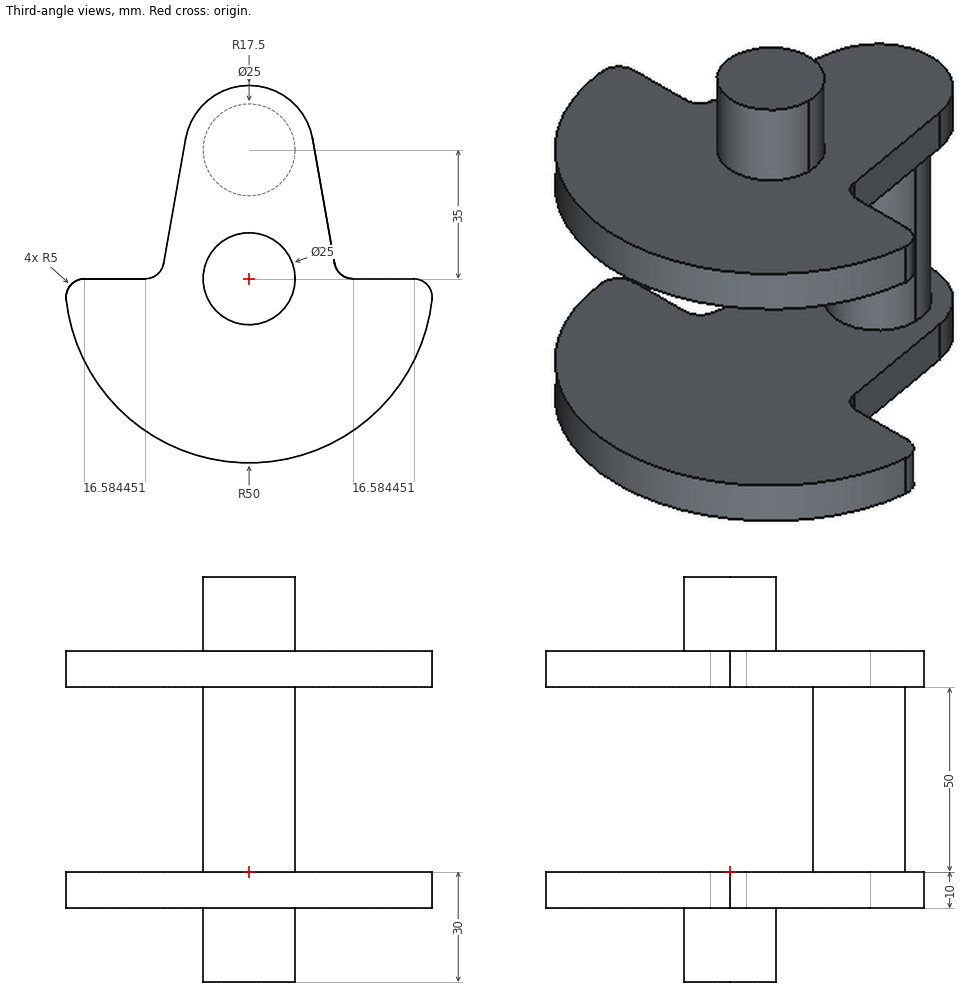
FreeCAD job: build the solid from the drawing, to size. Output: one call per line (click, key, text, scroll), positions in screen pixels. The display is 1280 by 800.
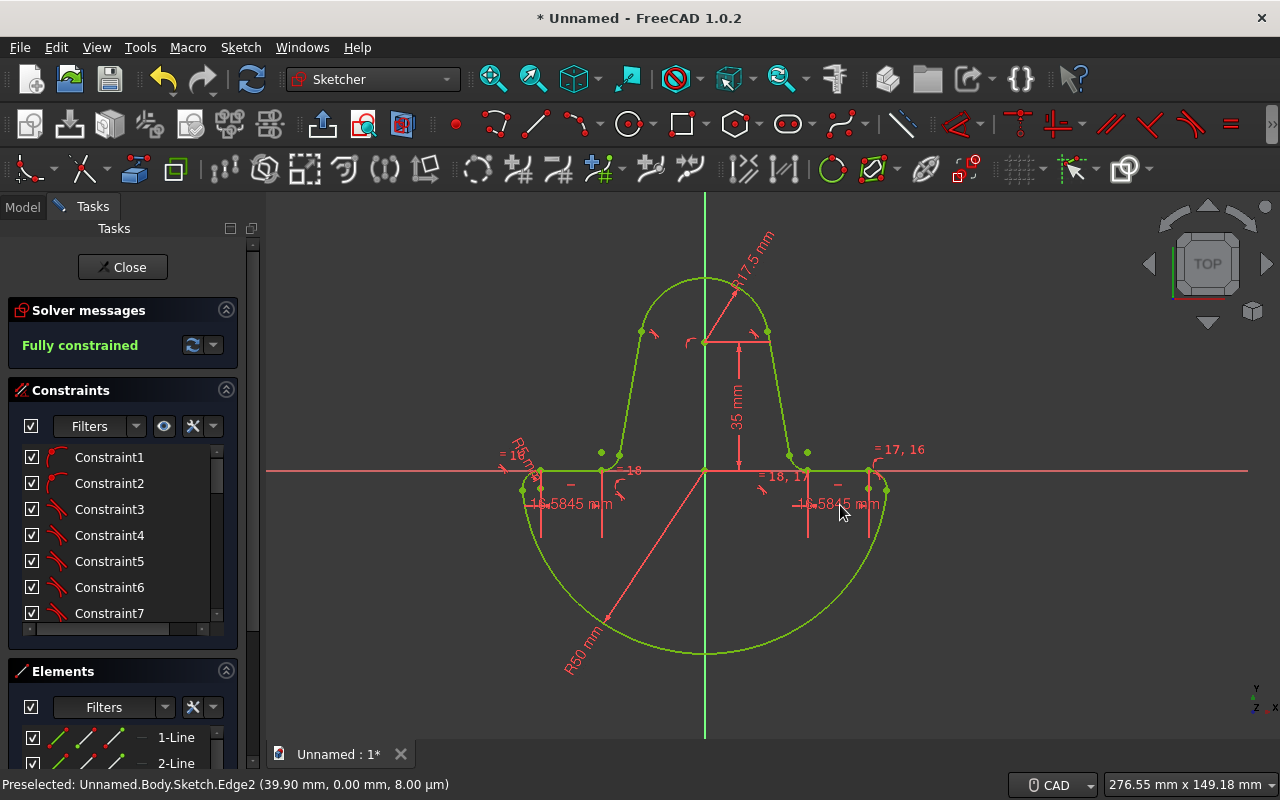
click(123, 267)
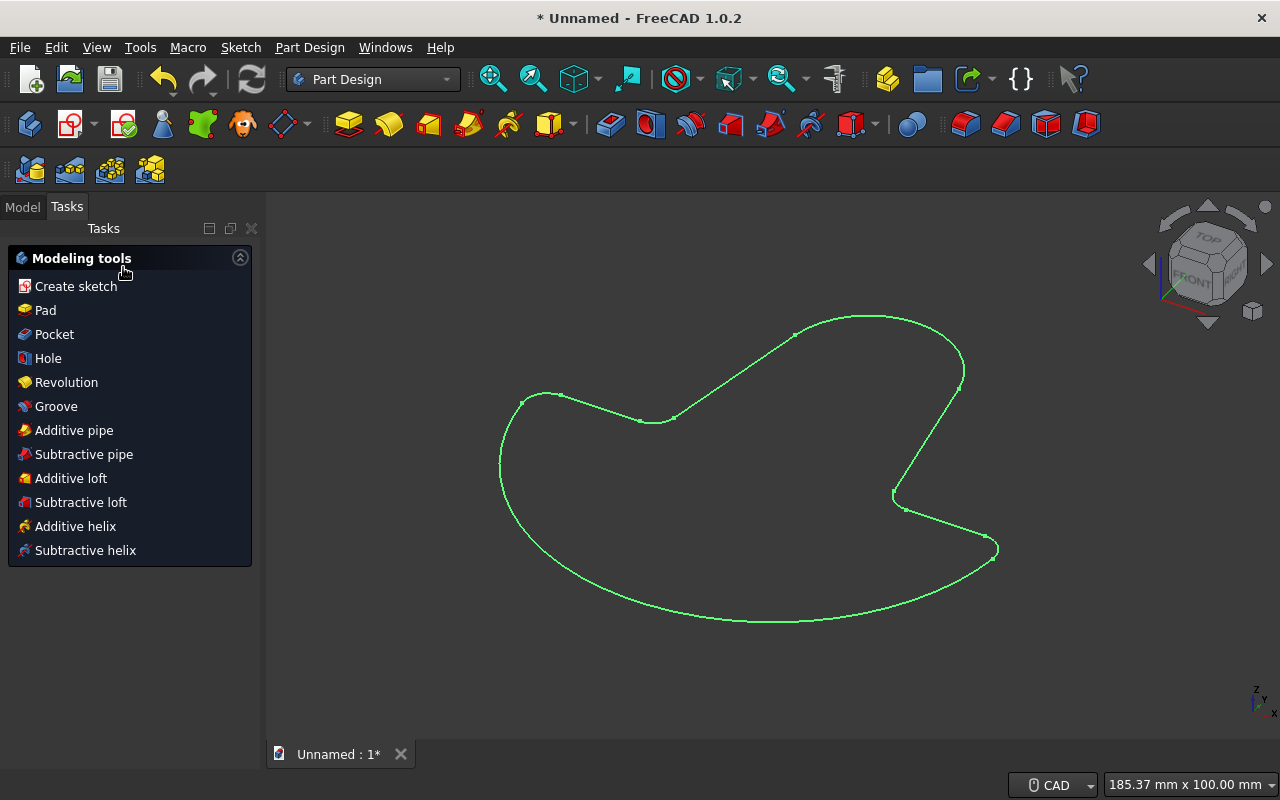
click(350, 124)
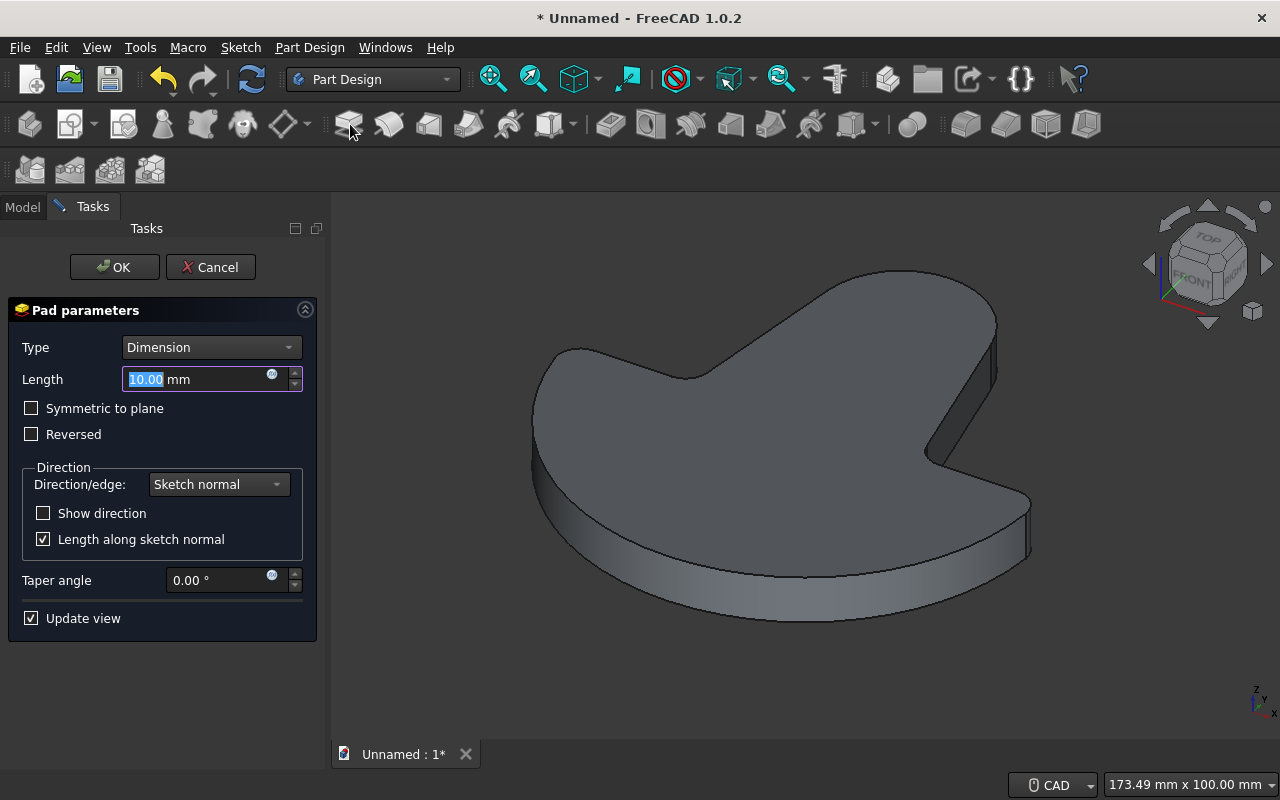
text(10)
key(Tab)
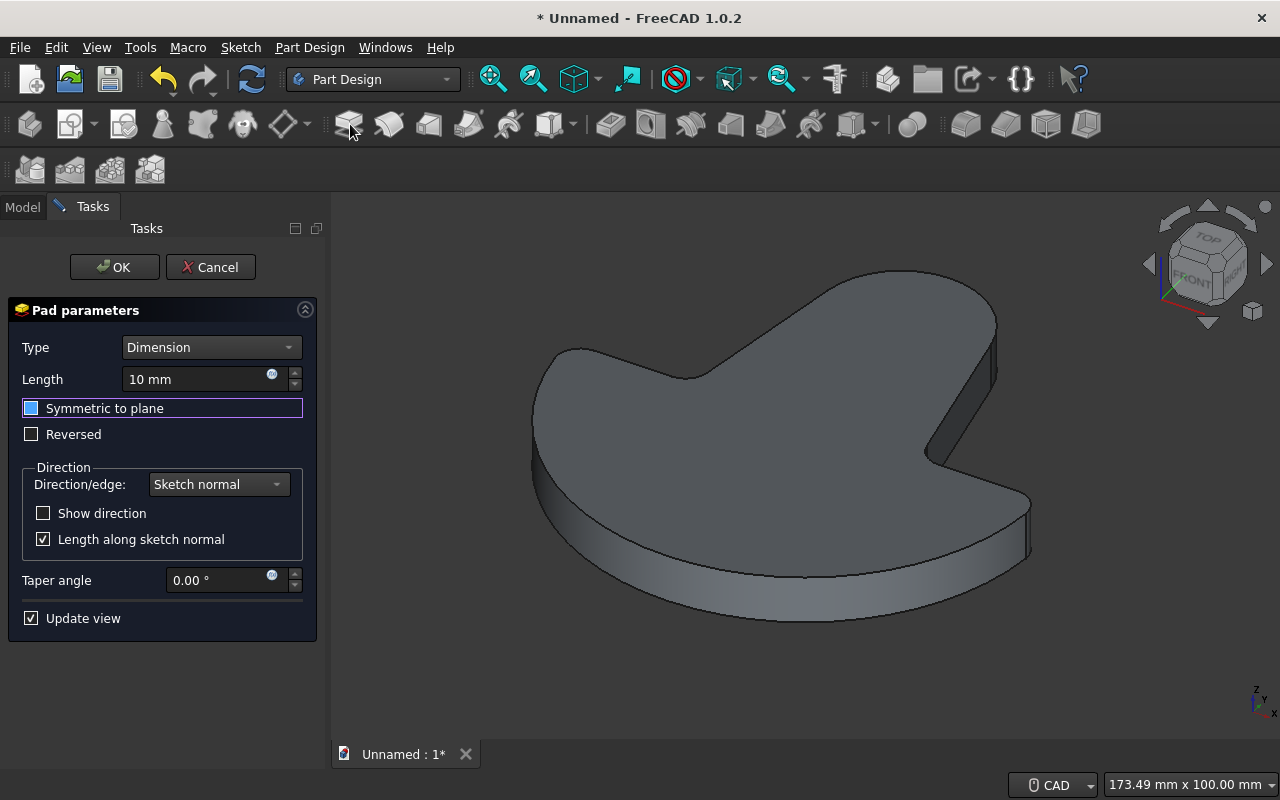
click(30, 434)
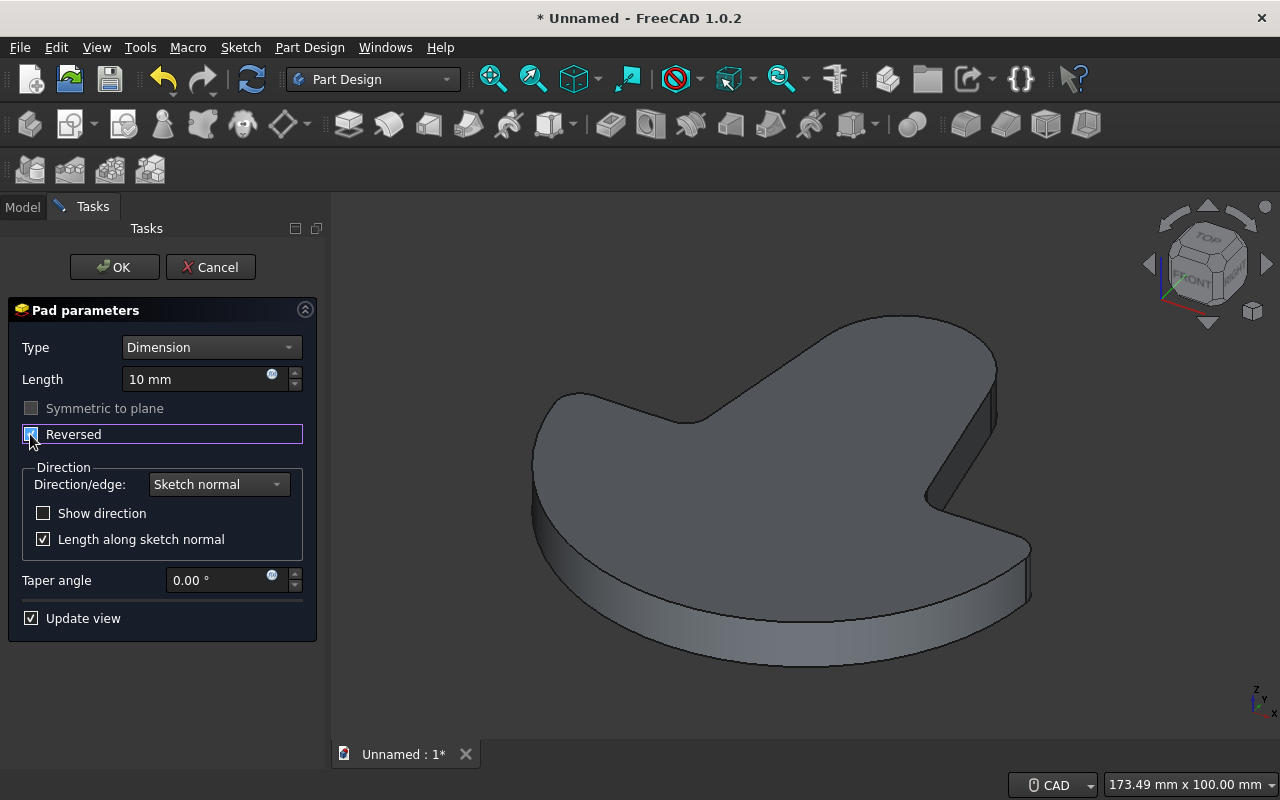
click(115, 267)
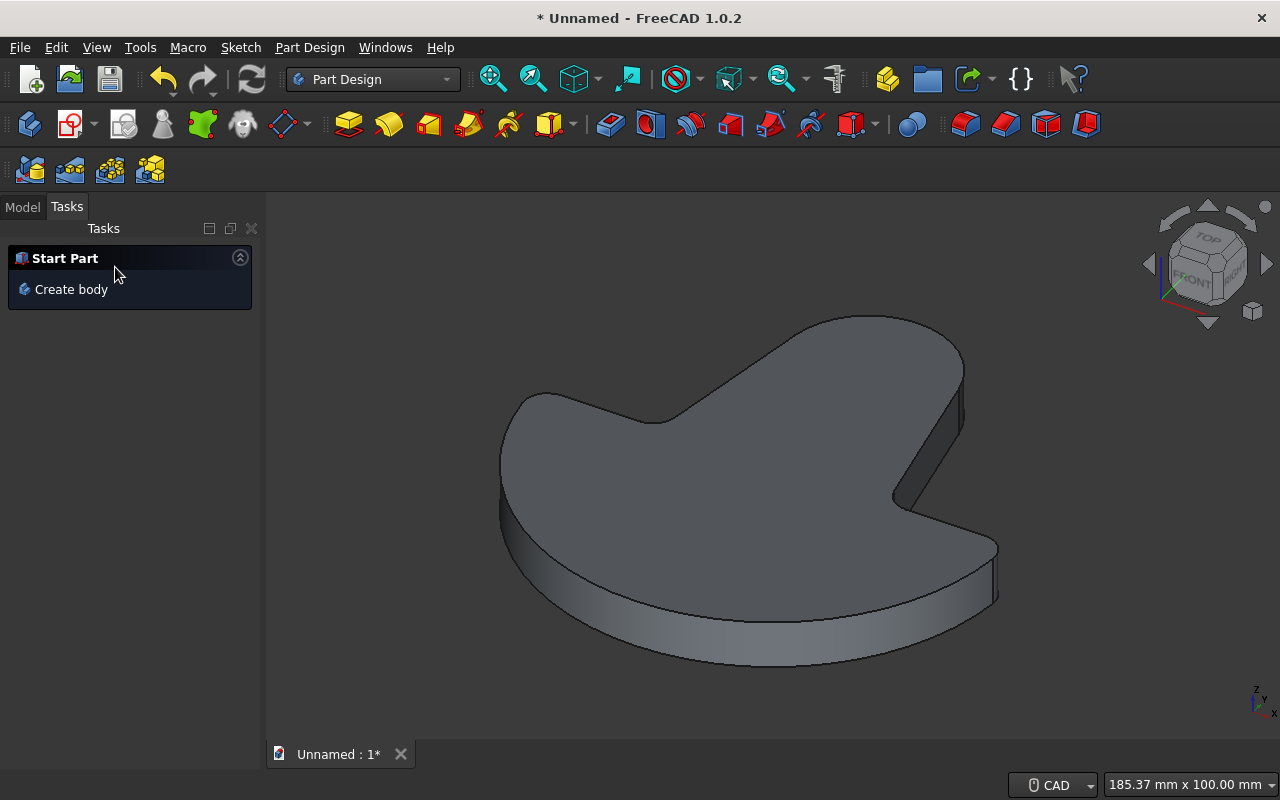
click(70, 124)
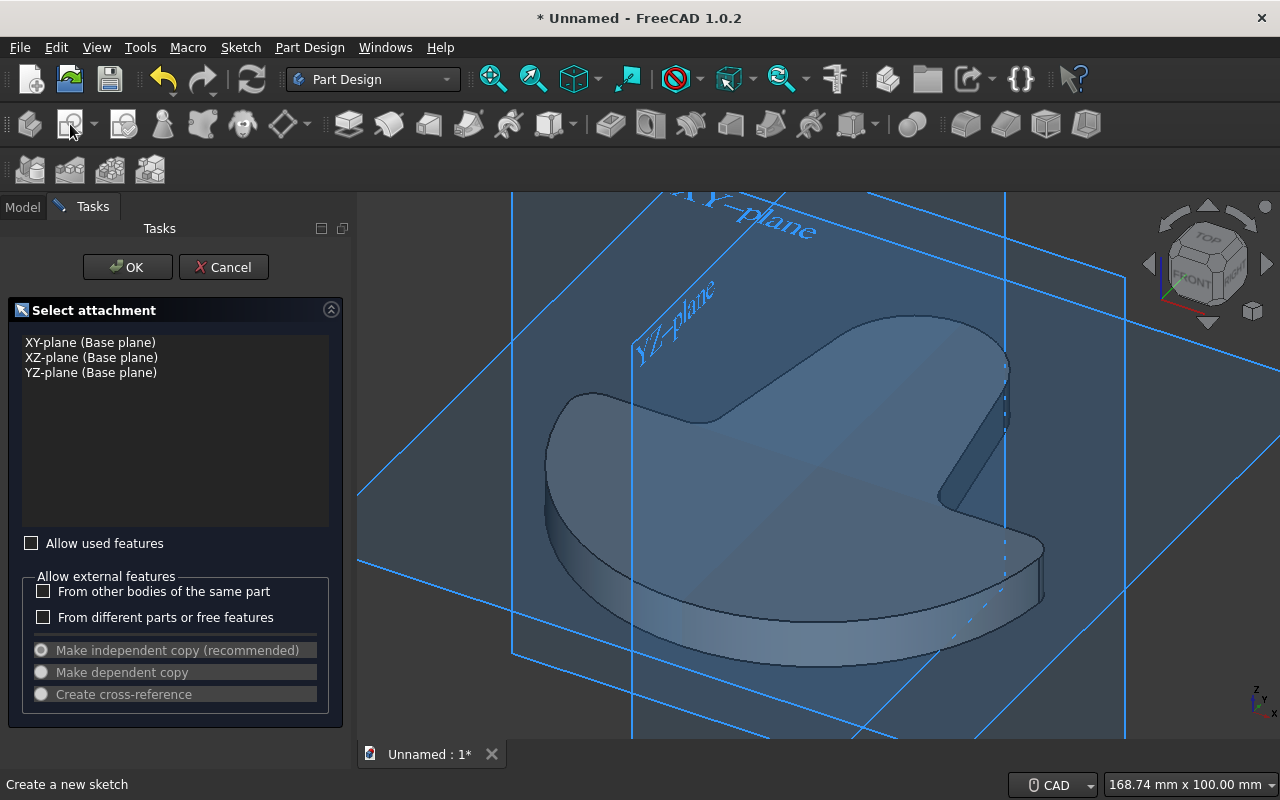
click(82, 342)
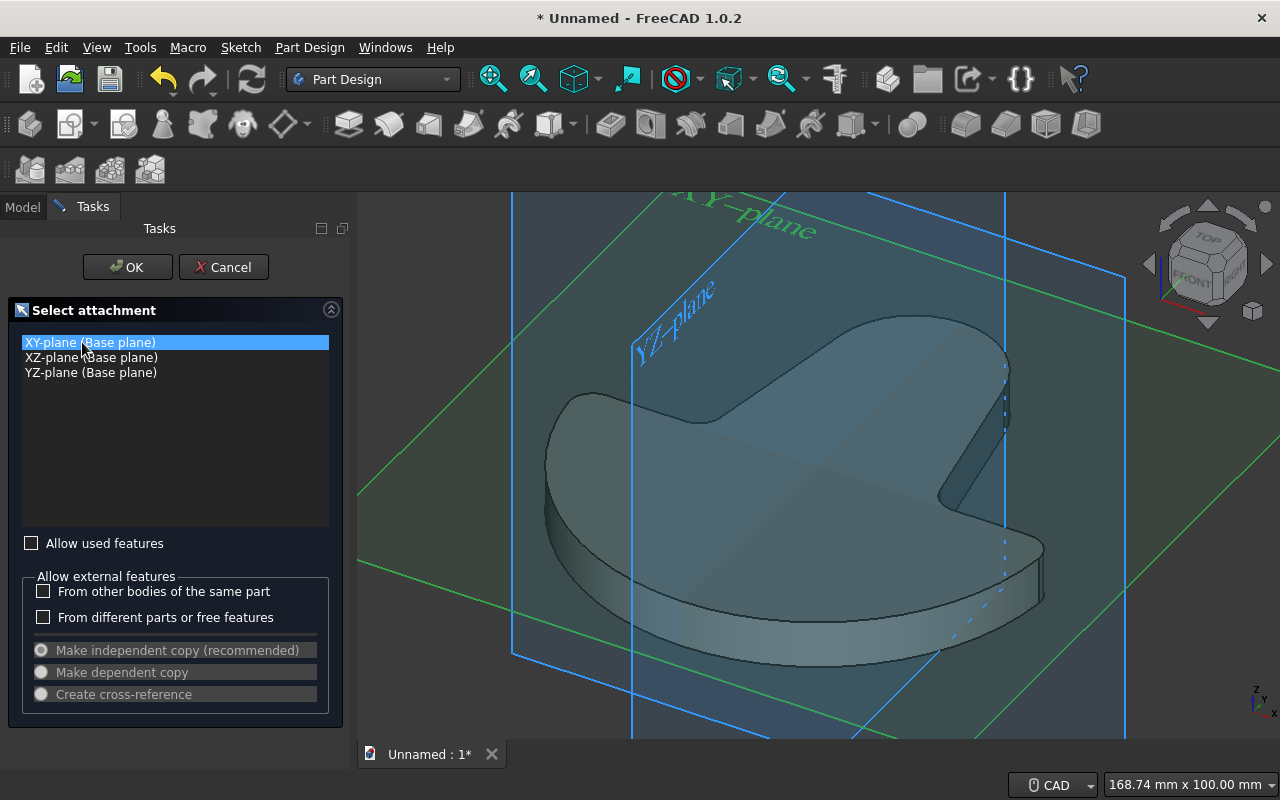
click(128, 267)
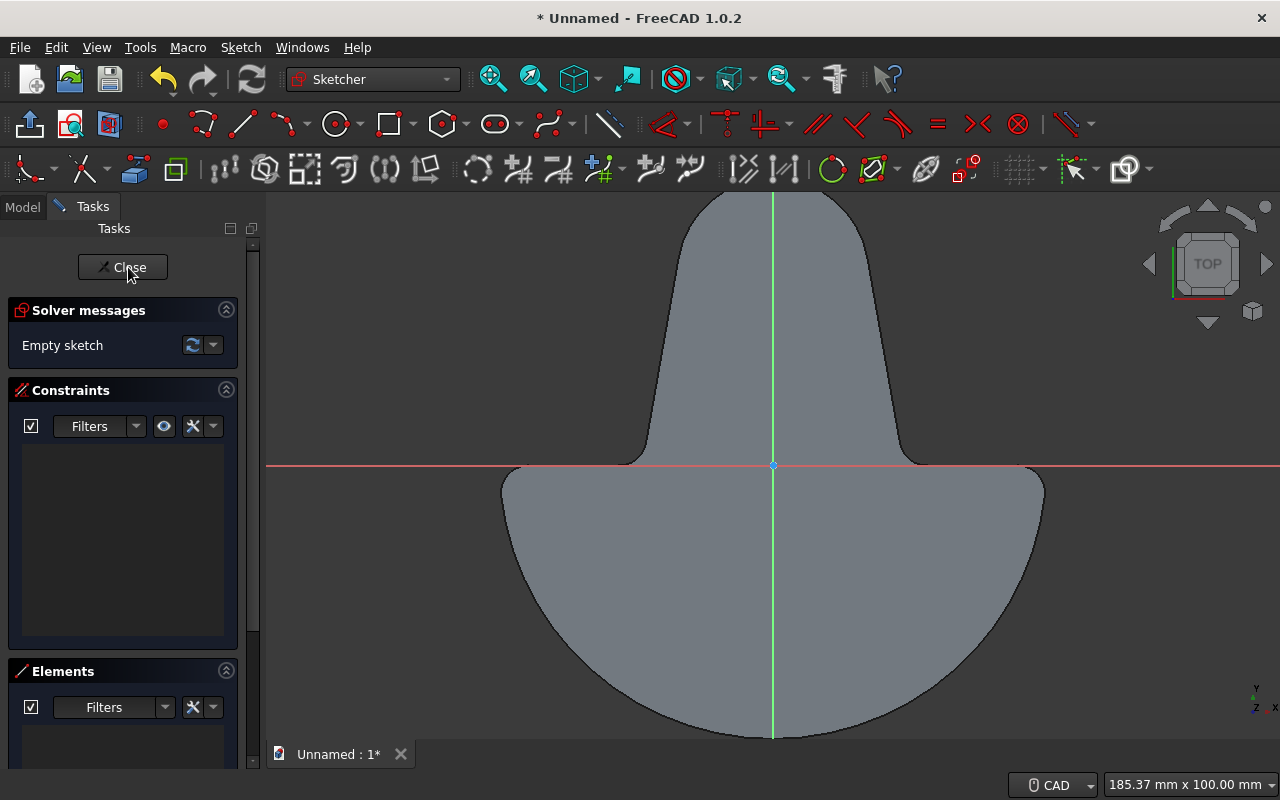
scroll(813, 466, up, 5)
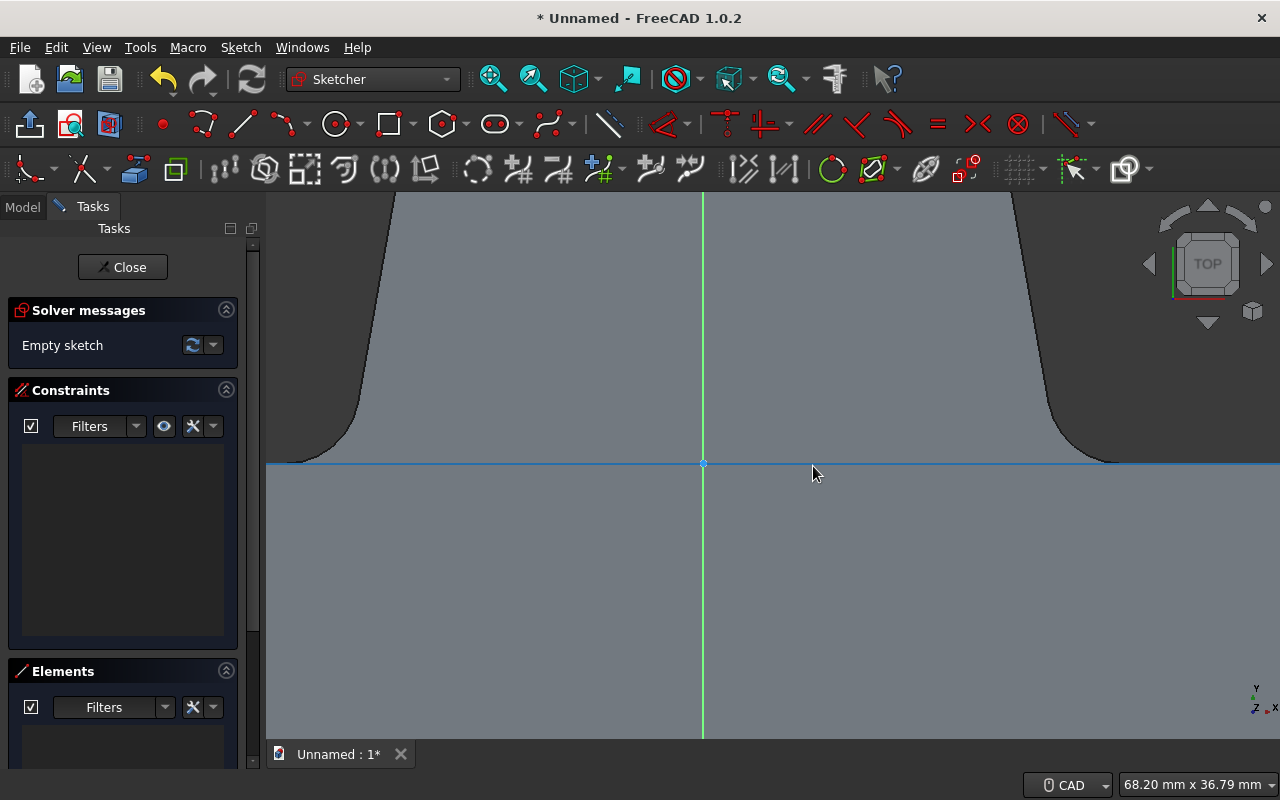
key(g)
key(c)